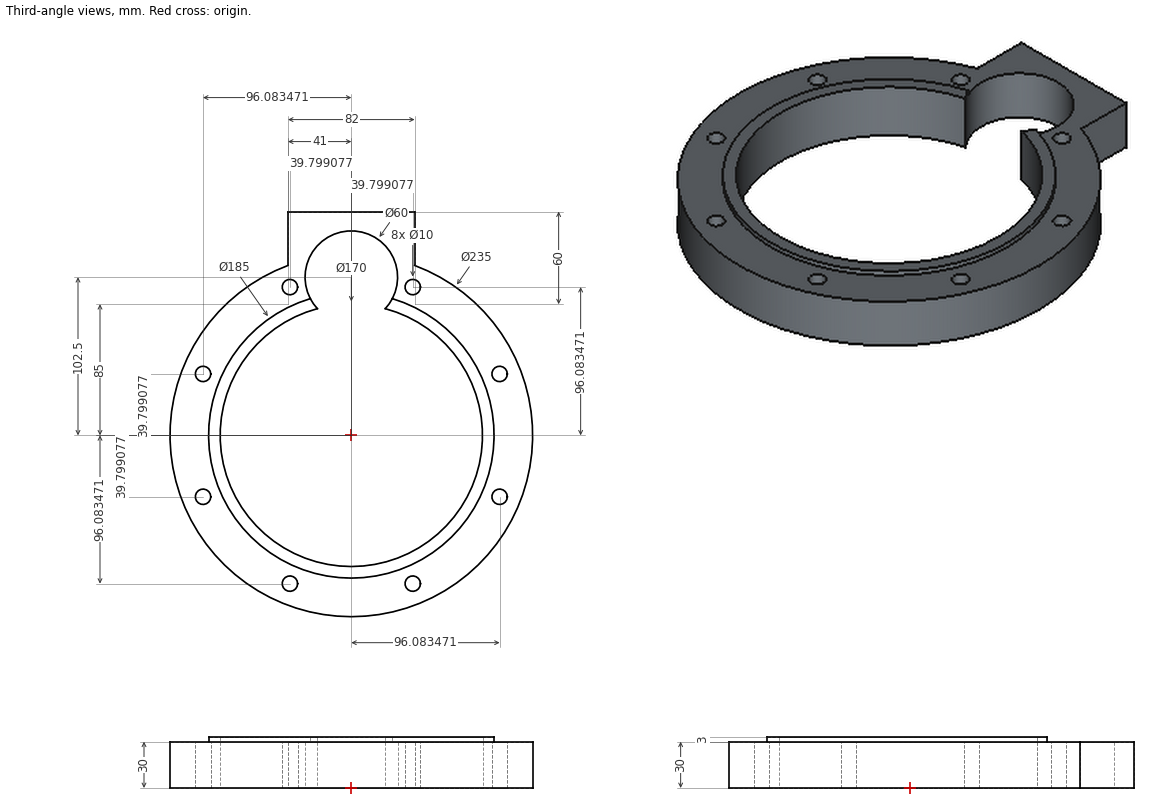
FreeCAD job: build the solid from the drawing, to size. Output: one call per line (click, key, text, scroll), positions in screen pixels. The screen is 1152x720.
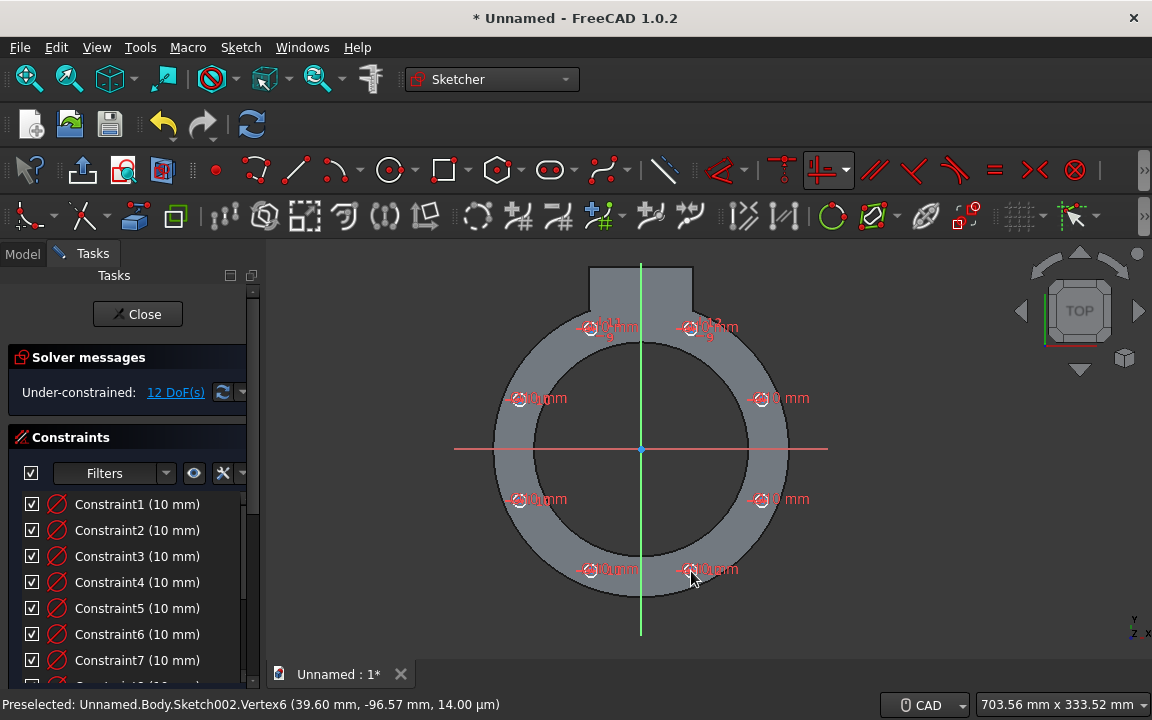
click(591, 571)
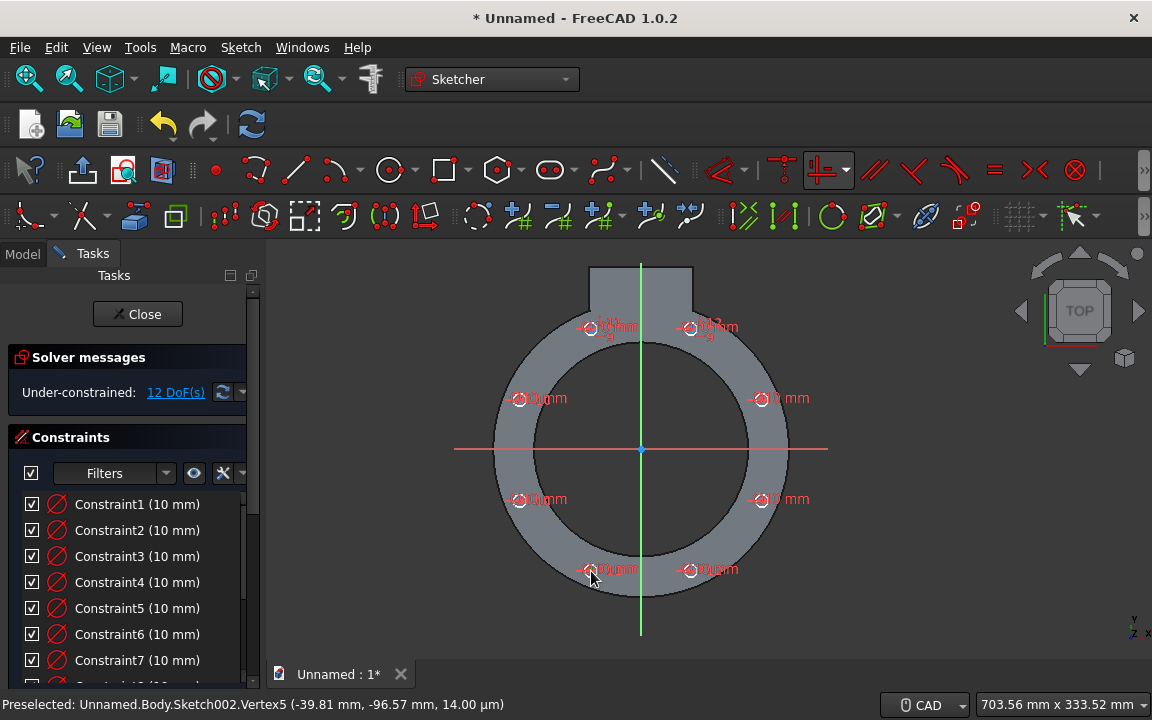
click(691, 571)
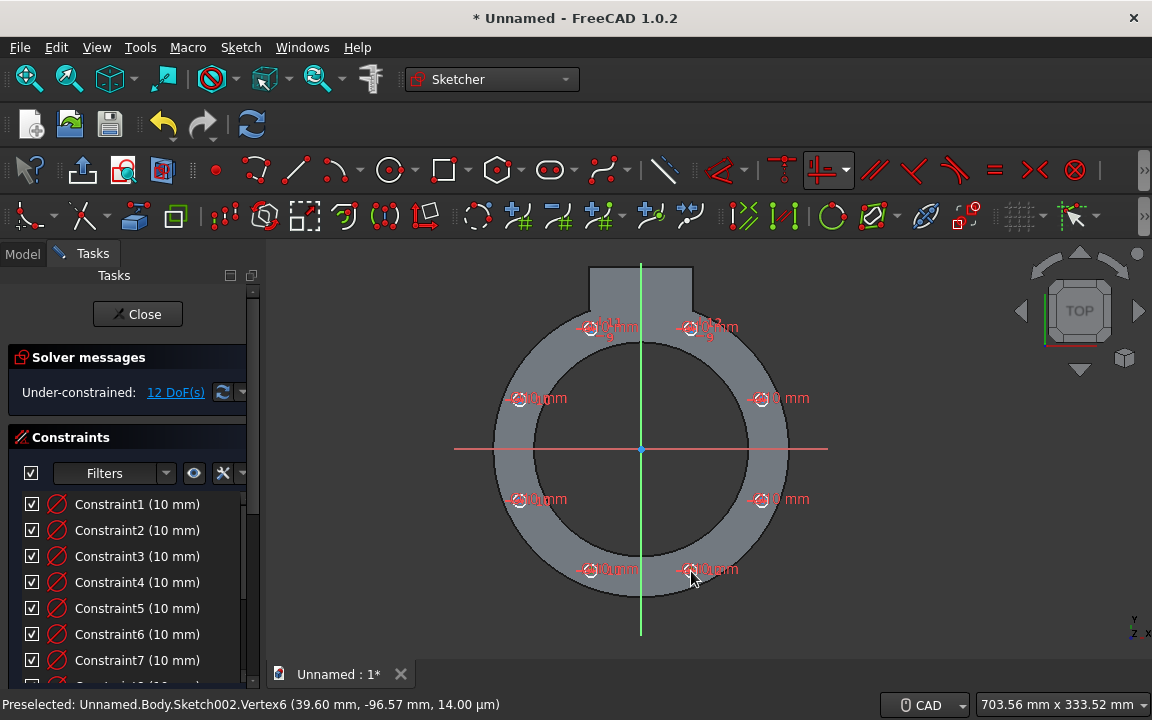
click(848, 170)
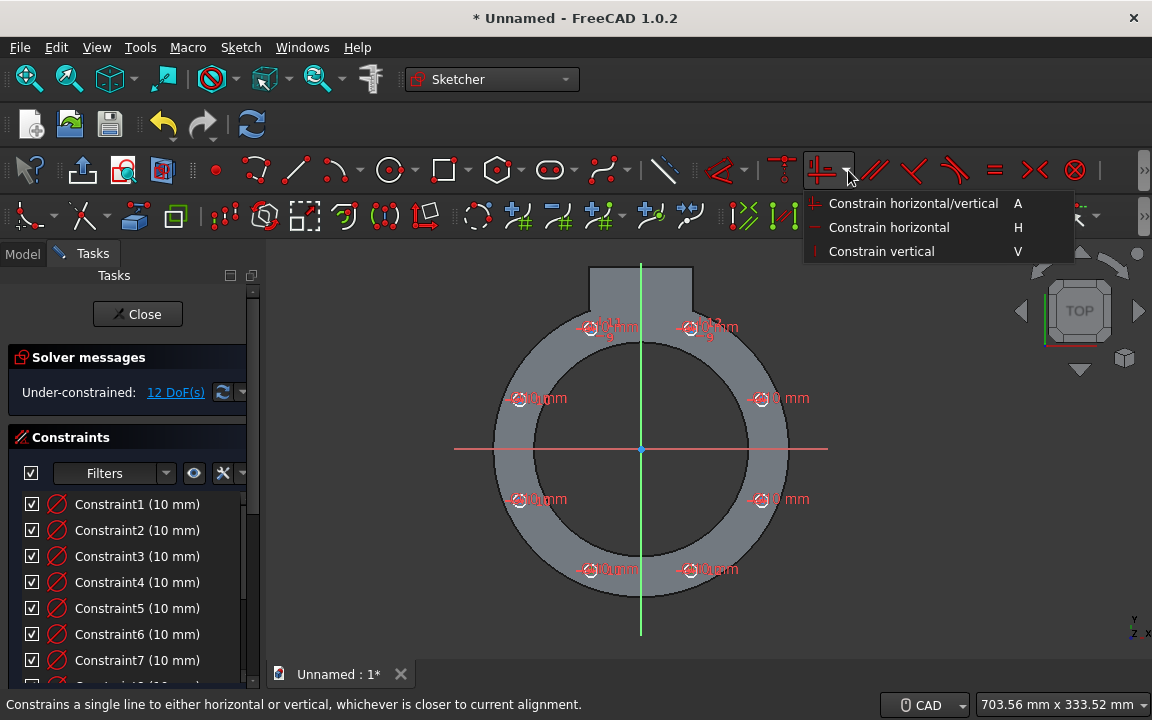
click(939, 227)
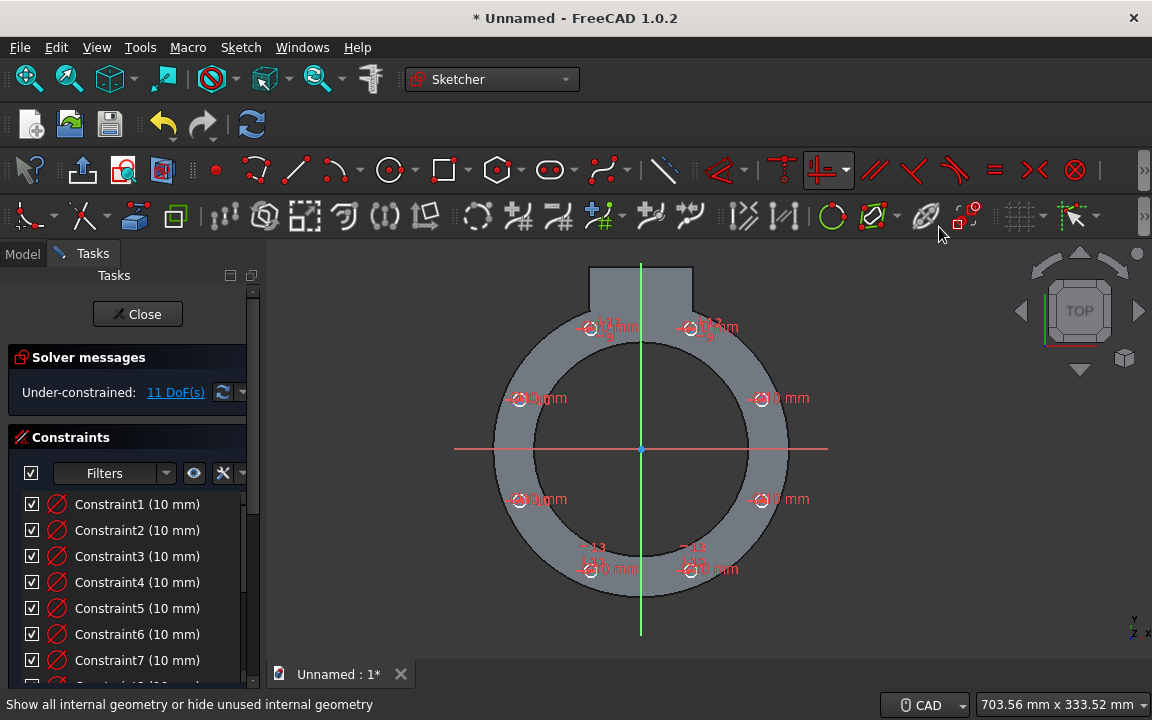
click(520, 501)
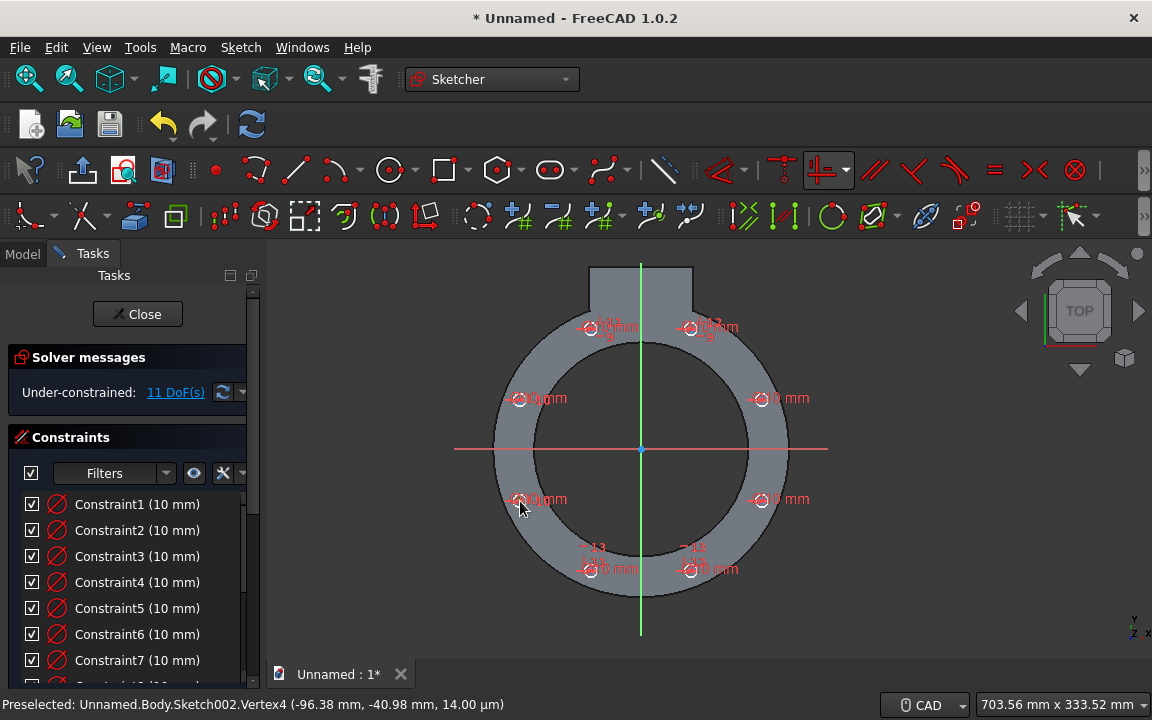
click(762, 501)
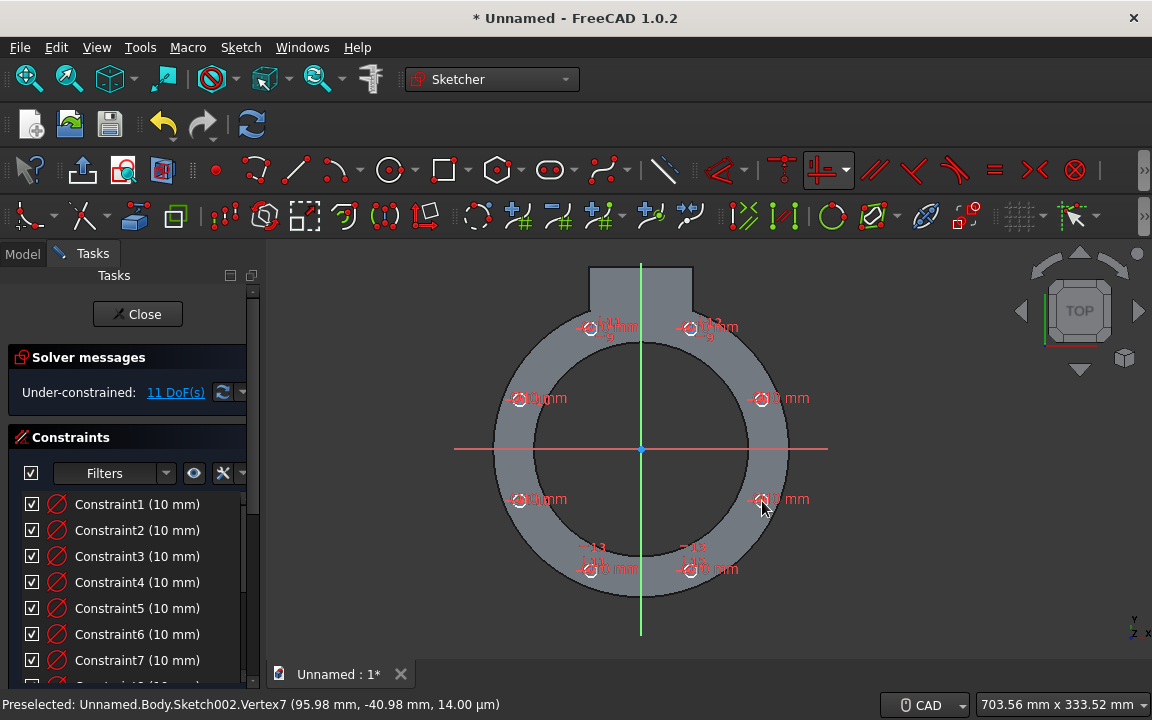
key(h)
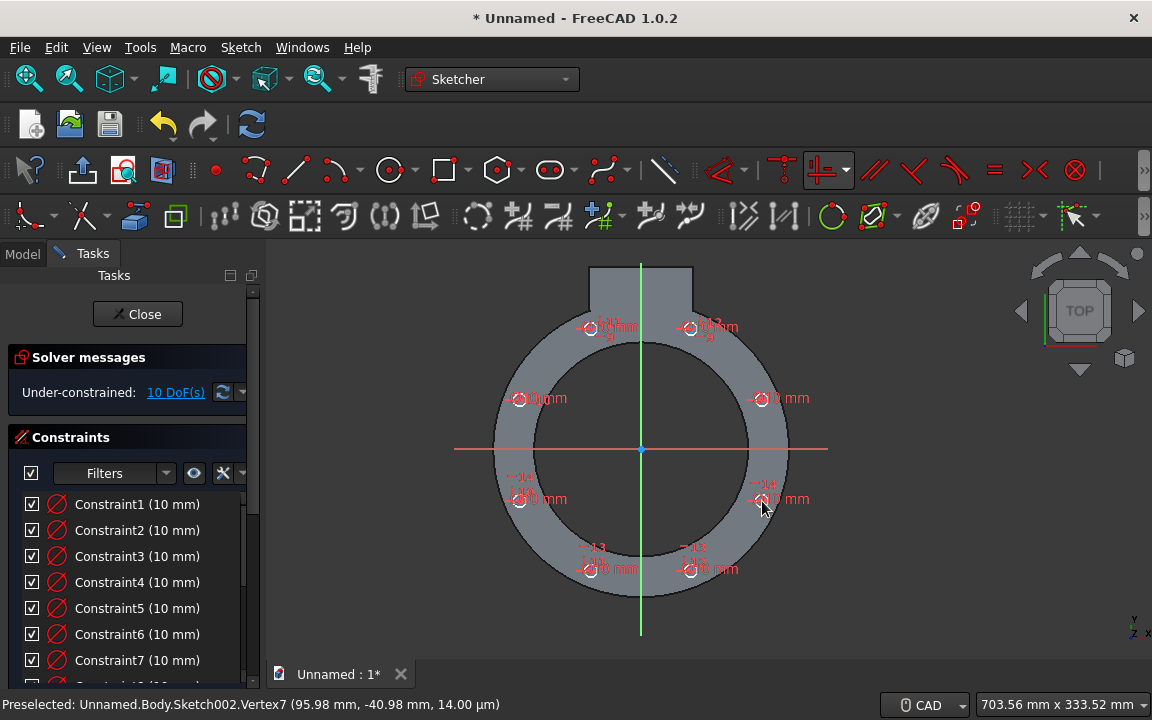
click(762, 501)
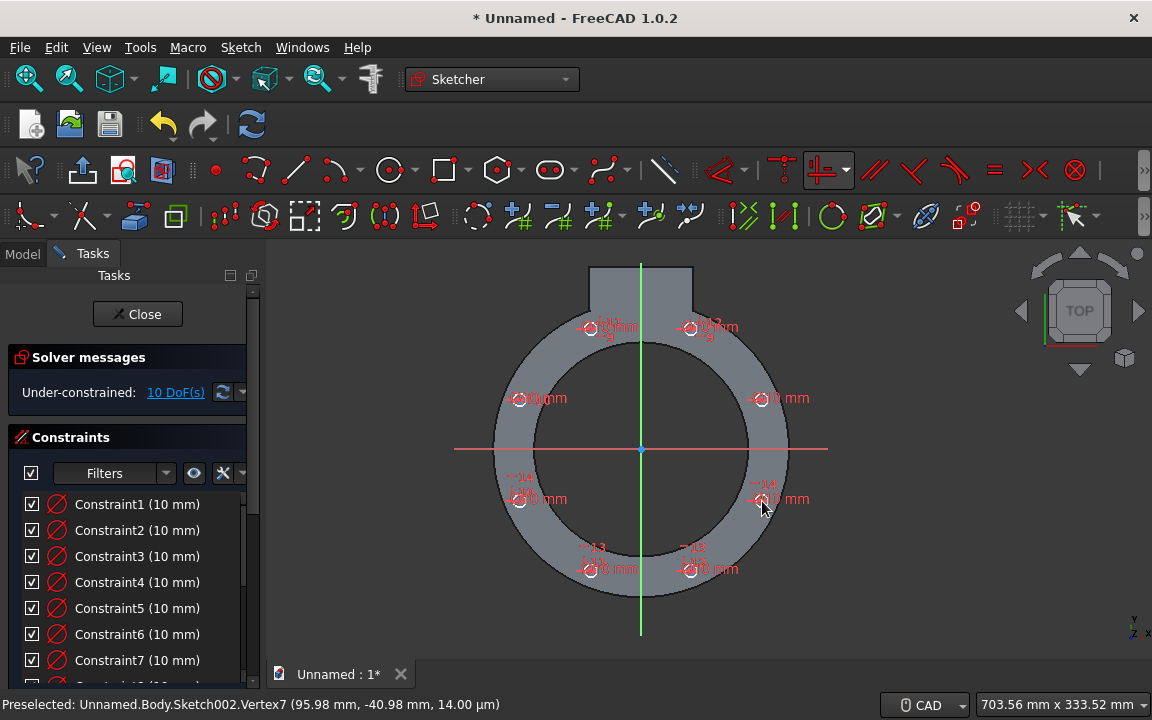
click(762, 400)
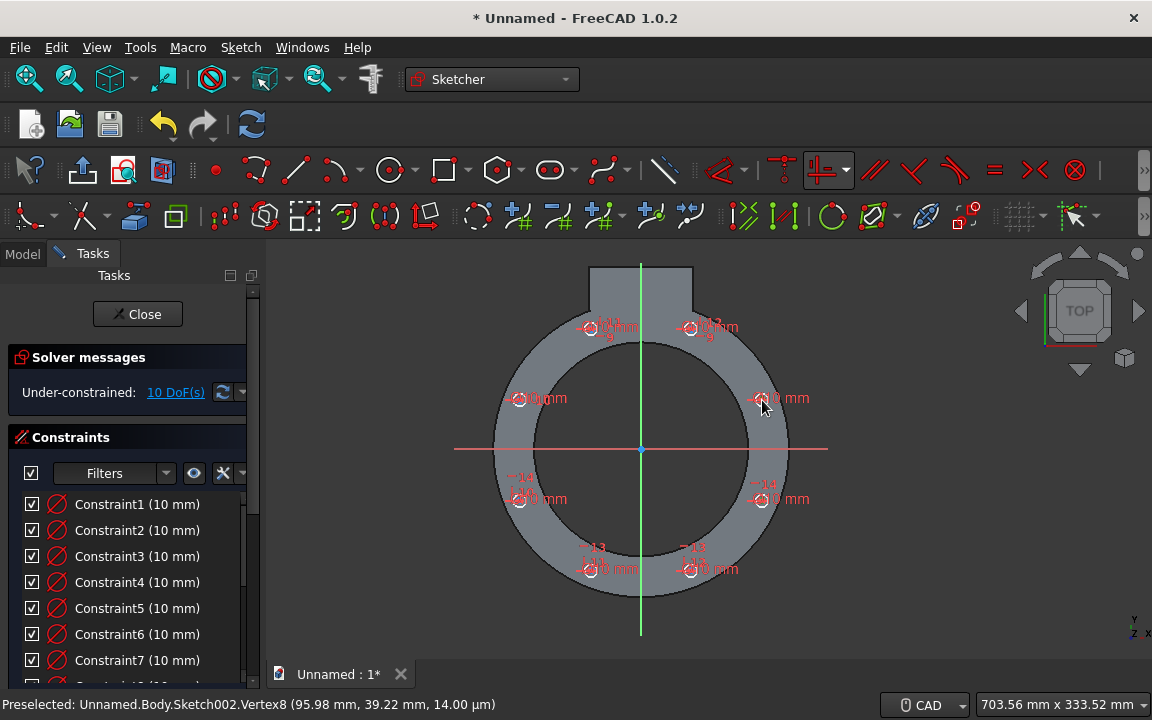
key(v)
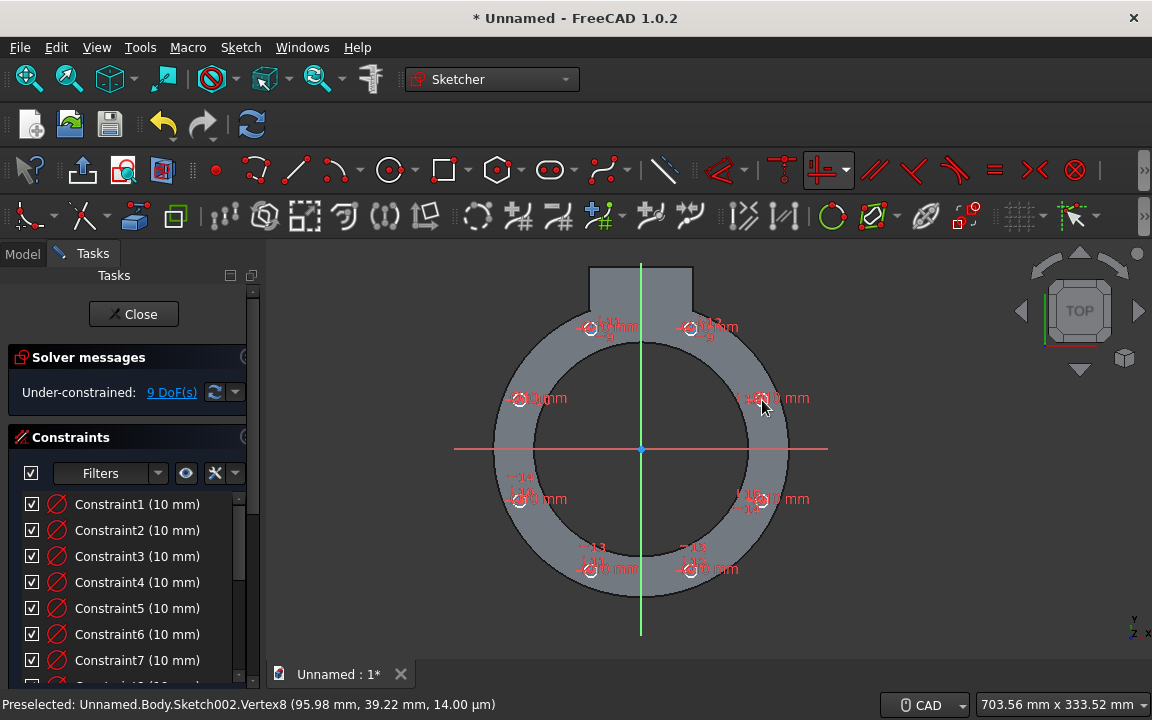
click(520, 400)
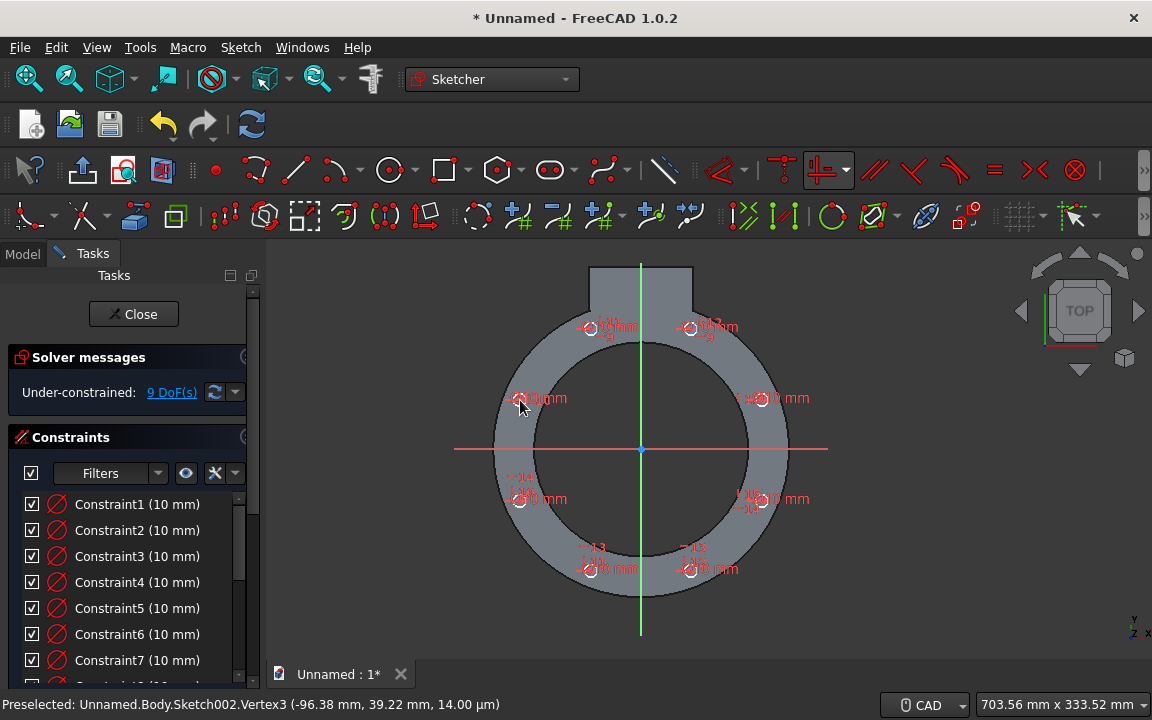
click(762, 400)